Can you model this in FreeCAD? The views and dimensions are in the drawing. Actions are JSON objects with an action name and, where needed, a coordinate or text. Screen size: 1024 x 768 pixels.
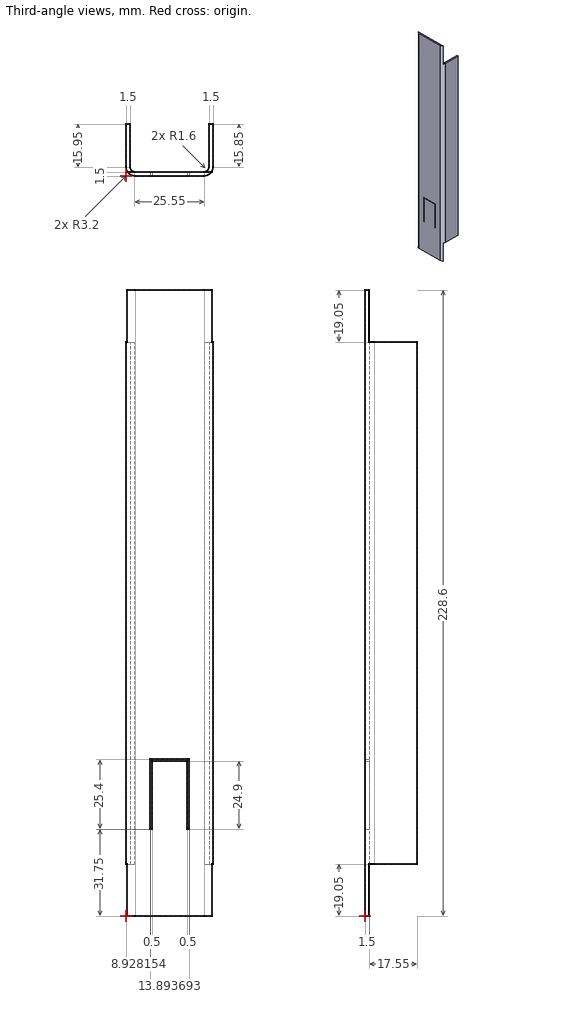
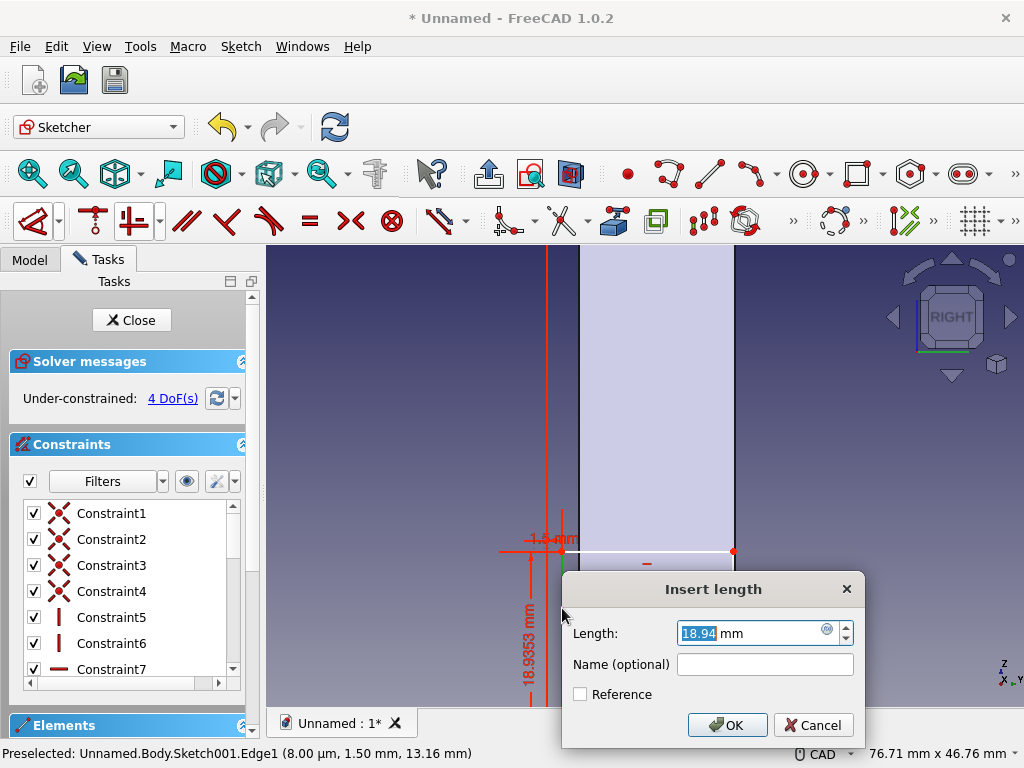
{"action": "type", "text": "19.05"}
{"action": "key", "text": "Return"}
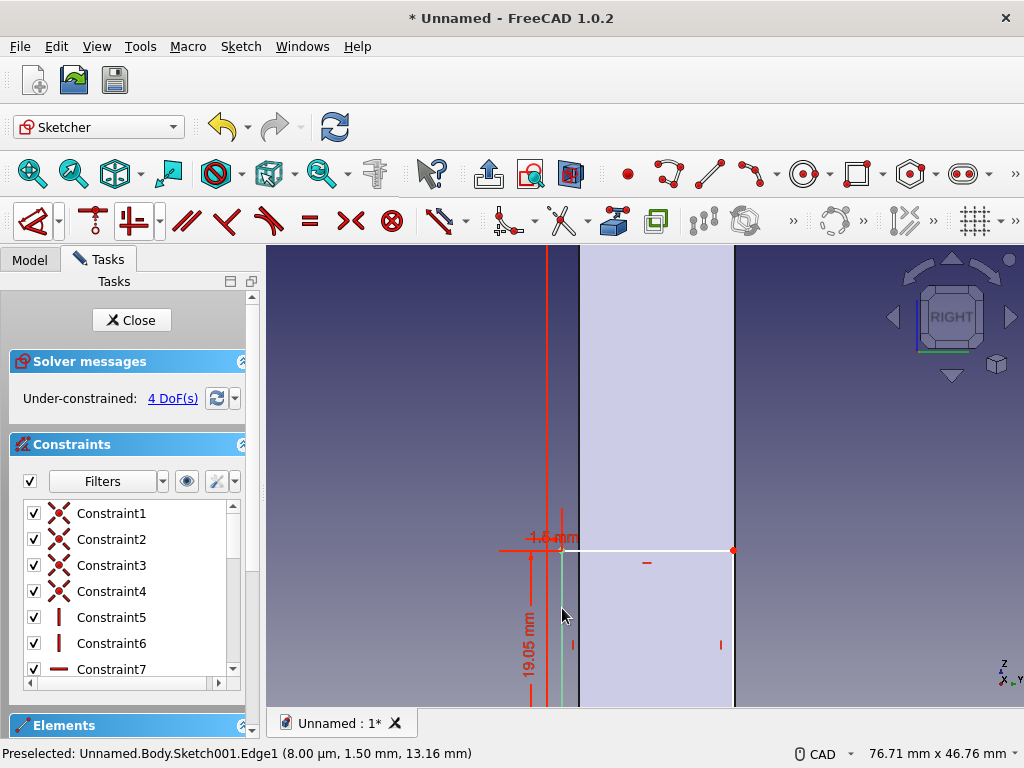
{"action": "scroll", "coordinate": [566, 612], "scroll_direction": "down", "scroll_amount": 10}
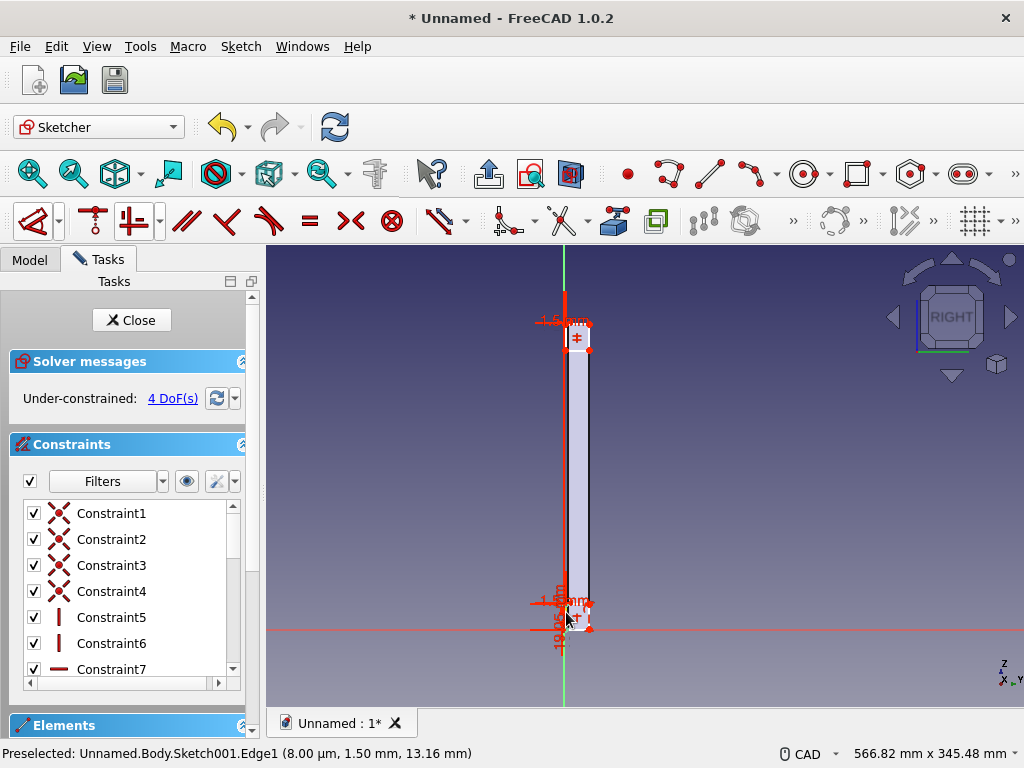
{"action": "scroll", "coordinate": [573, 630], "scroll_direction": "up", "scroll_amount": 4}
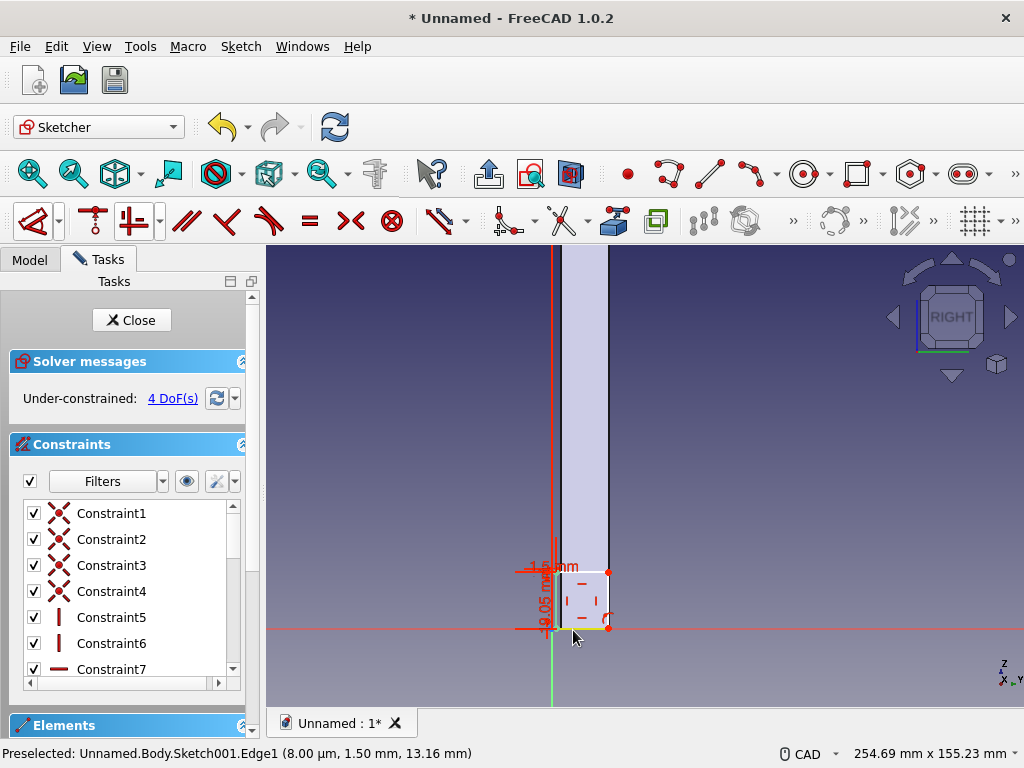
{"action": "left_click", "coordinate": [572, 629]}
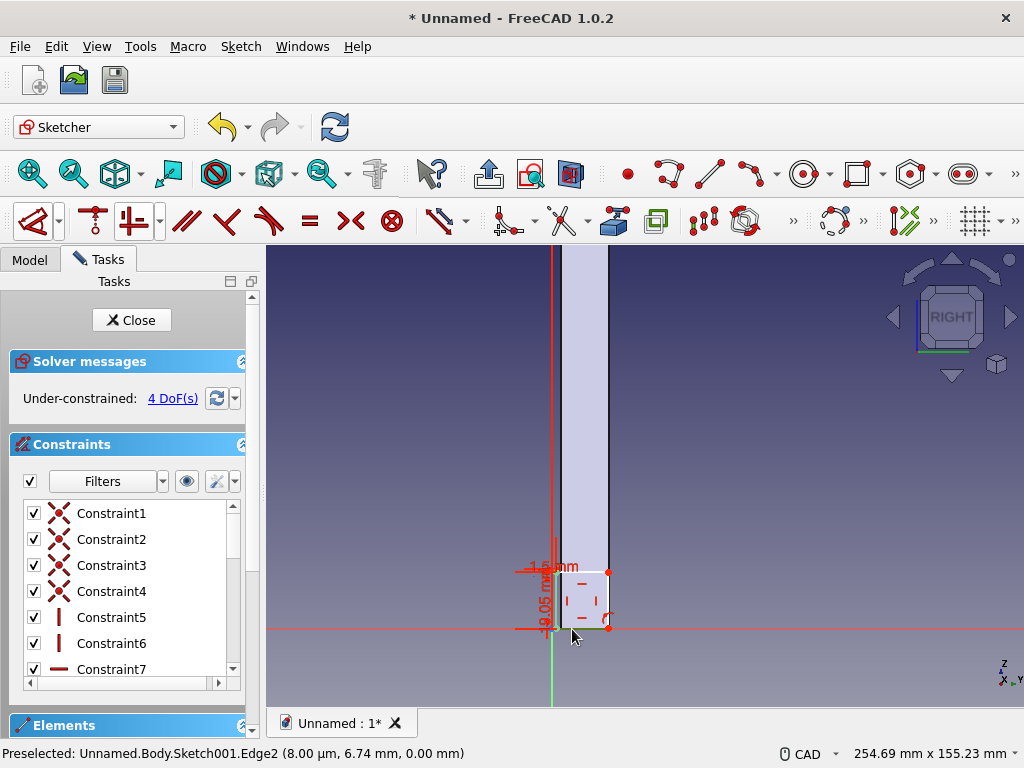
{"action": "key", "text": "l"}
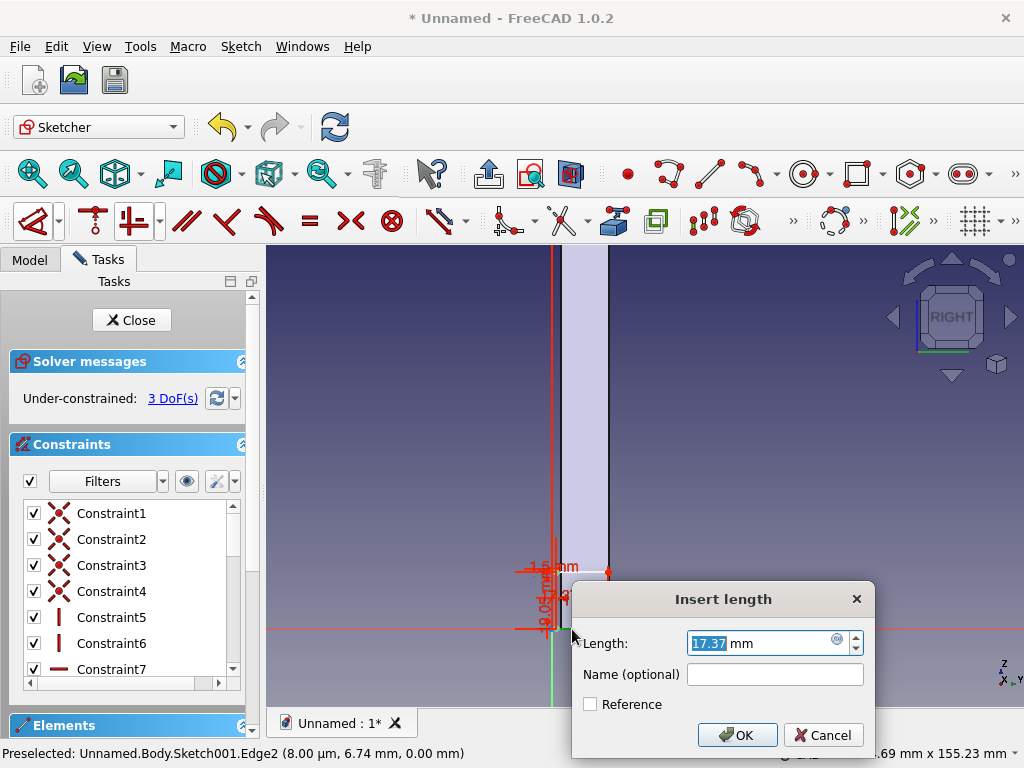
{"action": "type", "text": "17.55"}
{"action": "key", "text": "Return"}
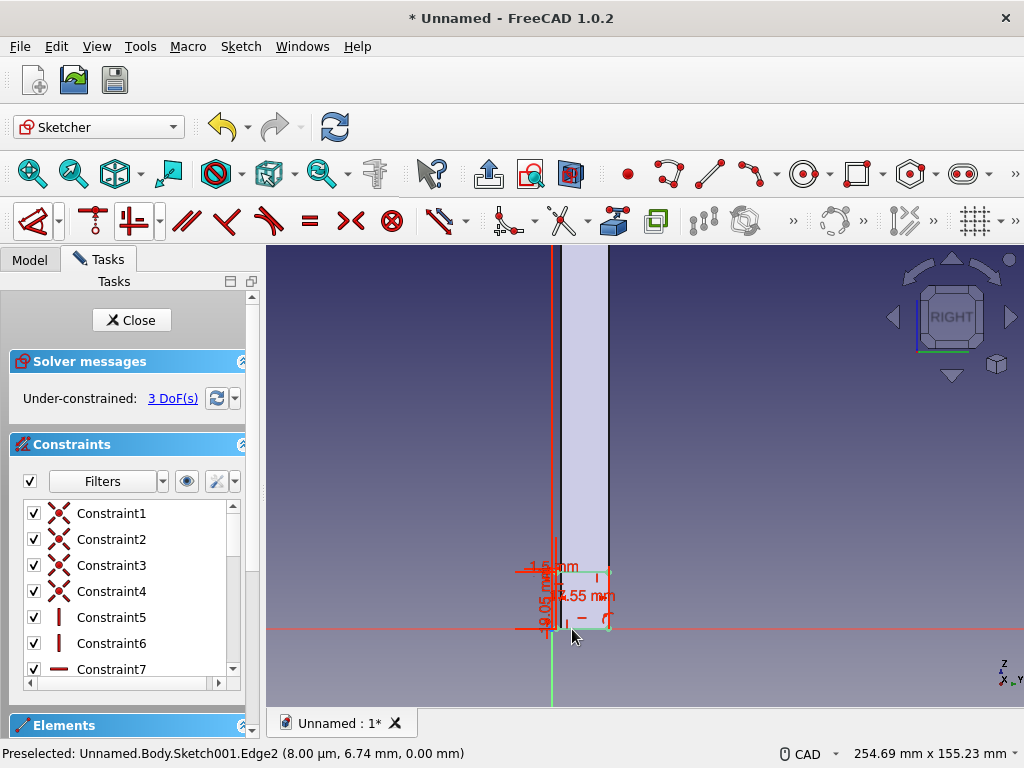
{"action": "scroll", "coordinate": [573, 629], "scroll_direction": "down", "scroll_amount": 4}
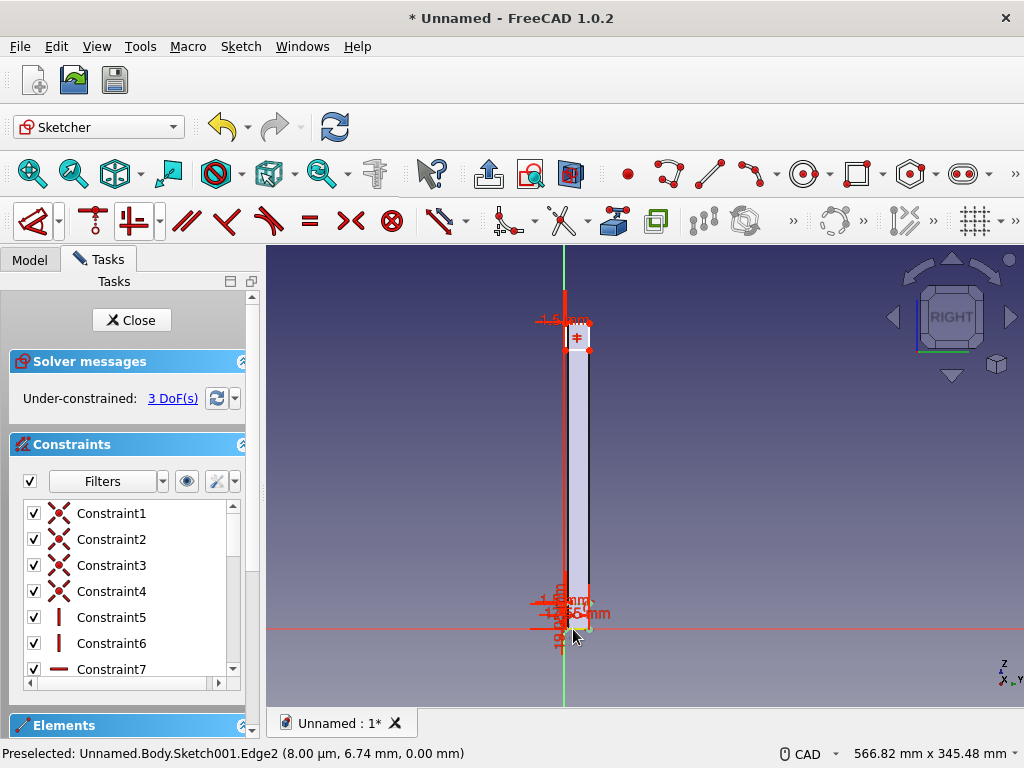
{"action": "scroll", "coordinate": [566, 332], "scroll_direction": "up", "scroll_amount": 10}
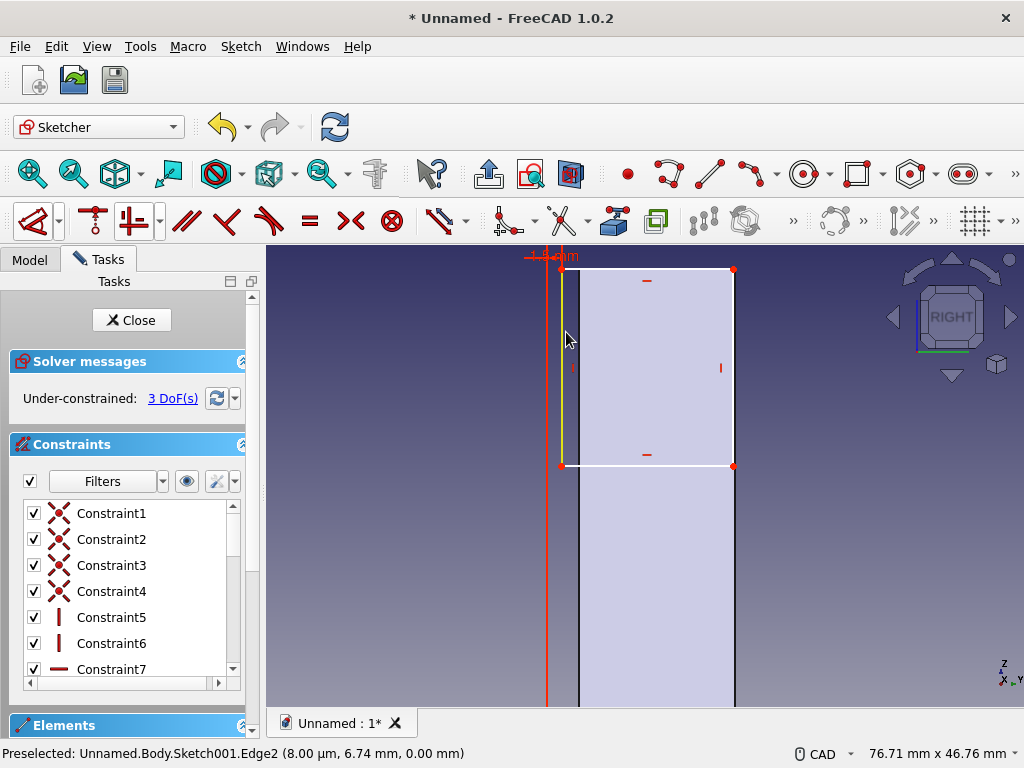
{"action": "left_click", "coordinate": [562, 328]}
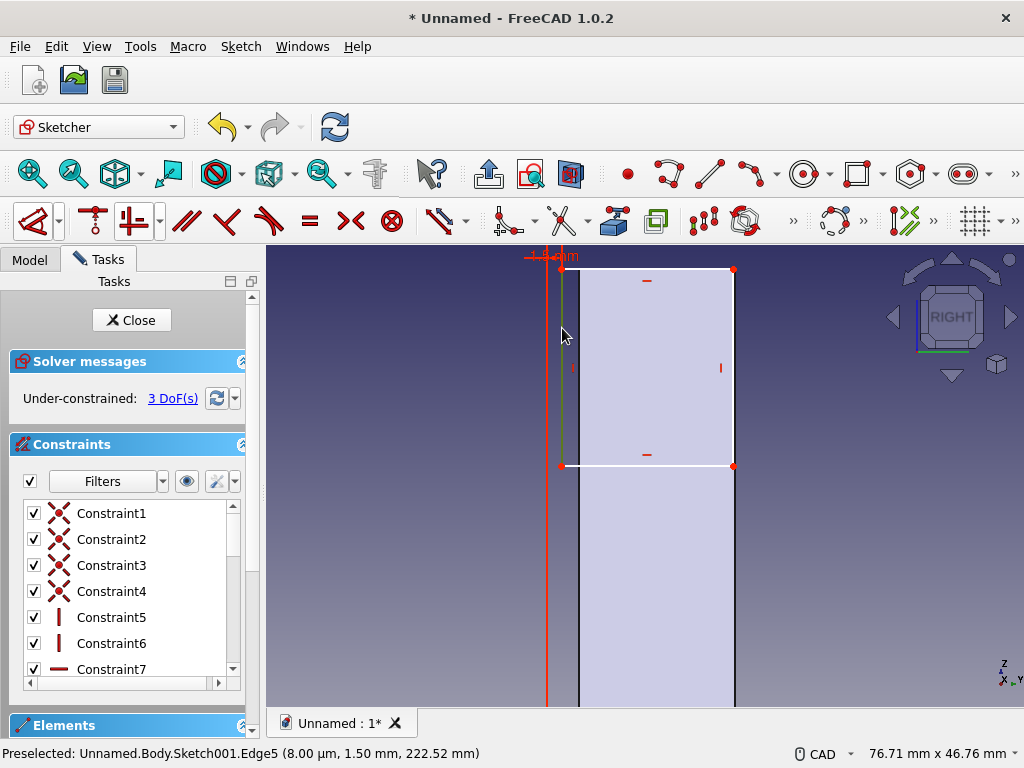
{"action": "key", "text": "i"}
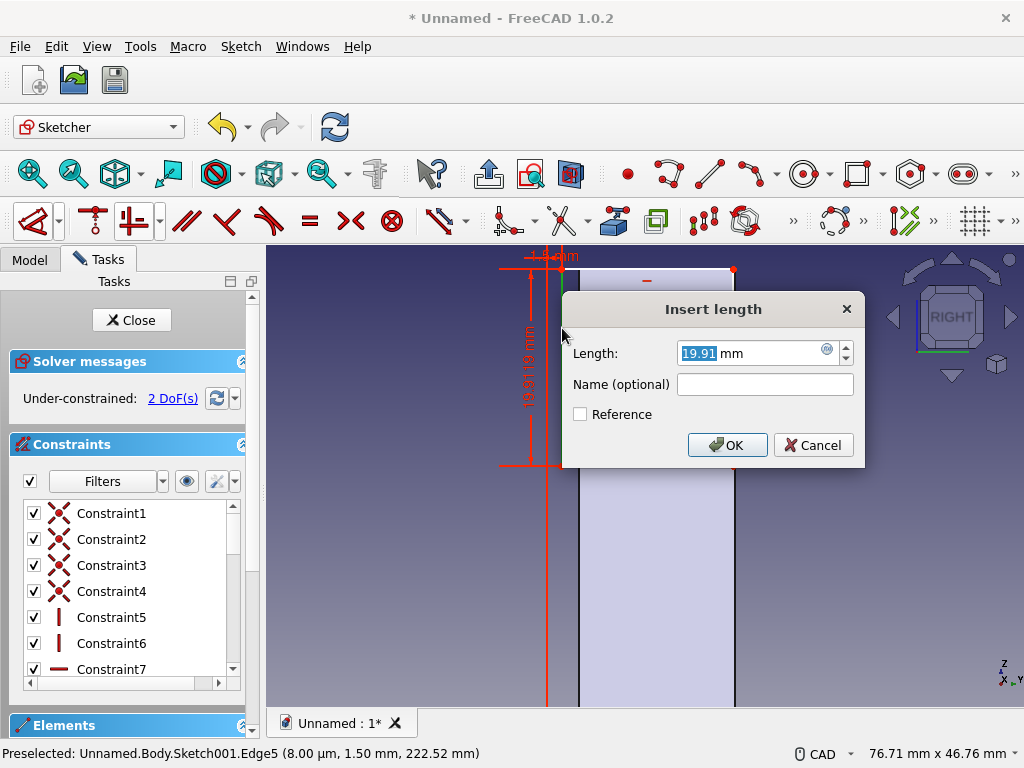
{"action": "type", "text": "19.05"}
{"action": "key", "text": "Return"}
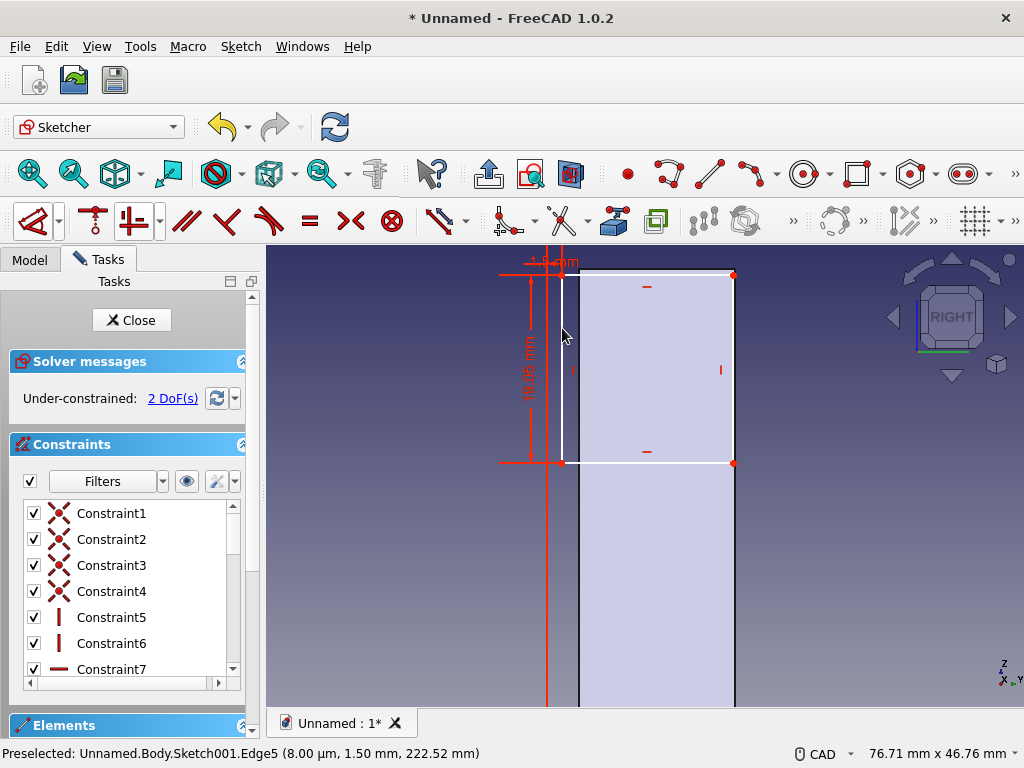
{"action": "scroll", "coordinate": [566, 332], "scroll_direction": "down", "scroll_amount": 10}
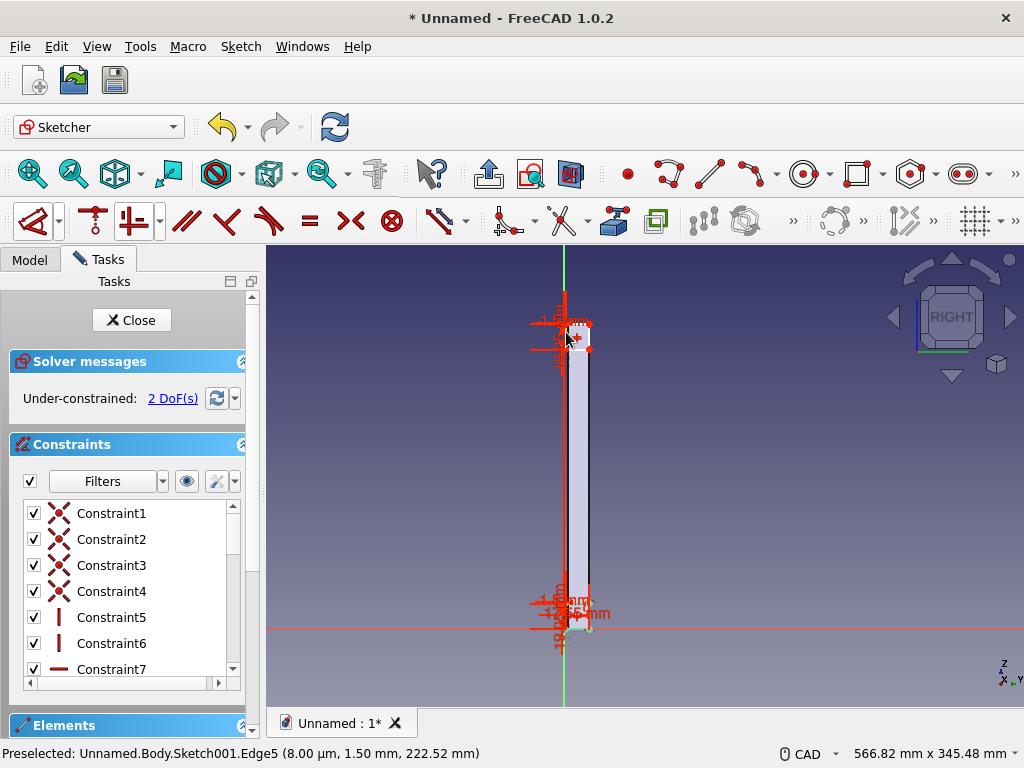
{"action": "scroll", "coordinate": [573, 350], "scroll_direction": "up", "scroll_amount": 4}